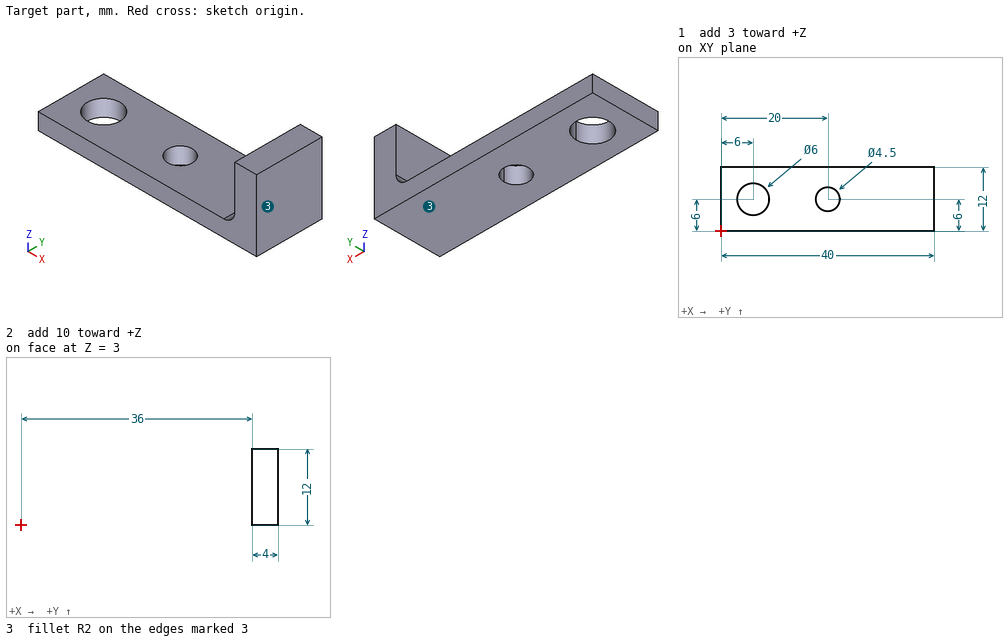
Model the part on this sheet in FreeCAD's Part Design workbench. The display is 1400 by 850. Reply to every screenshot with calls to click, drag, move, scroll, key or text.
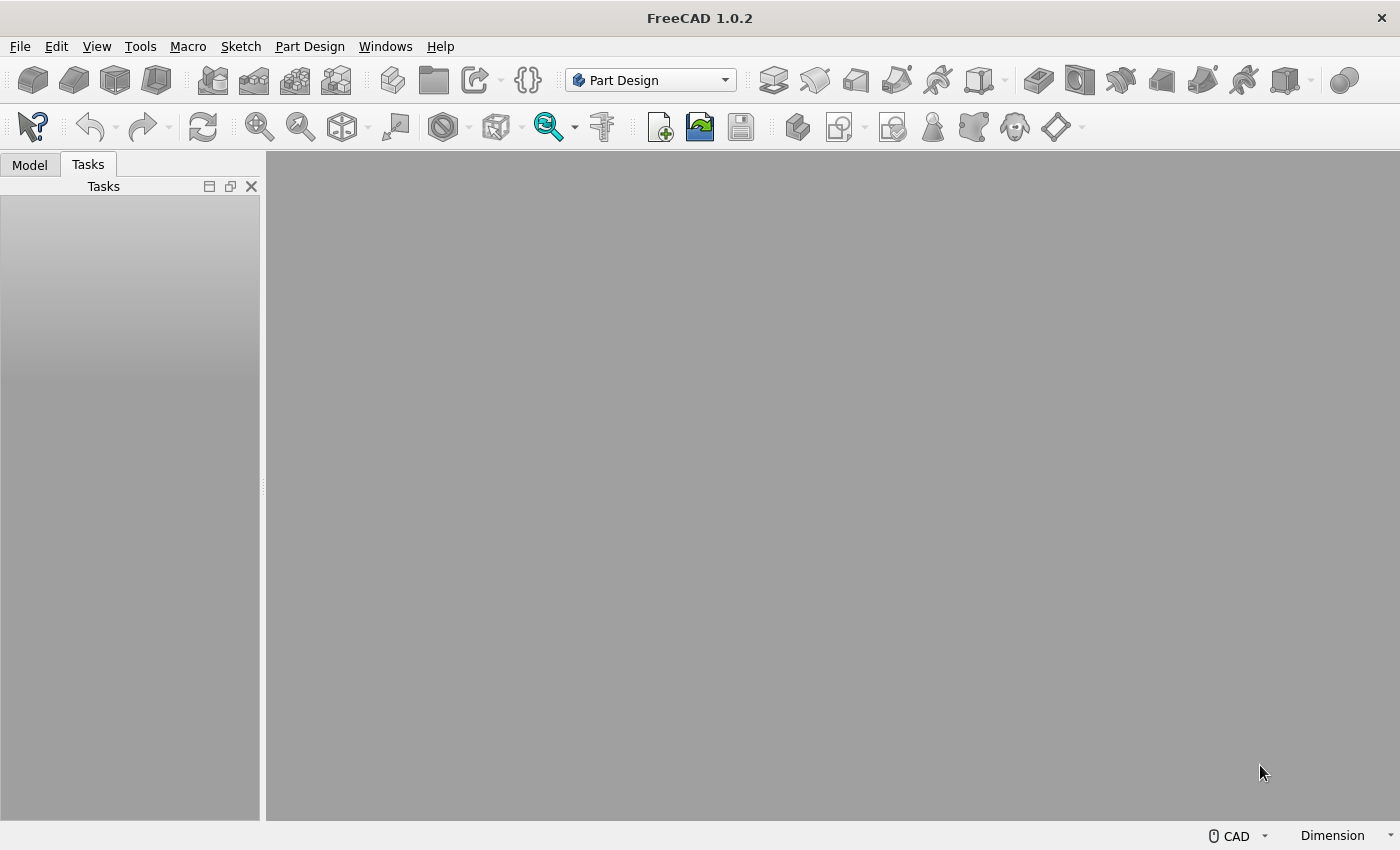
click(659, 128)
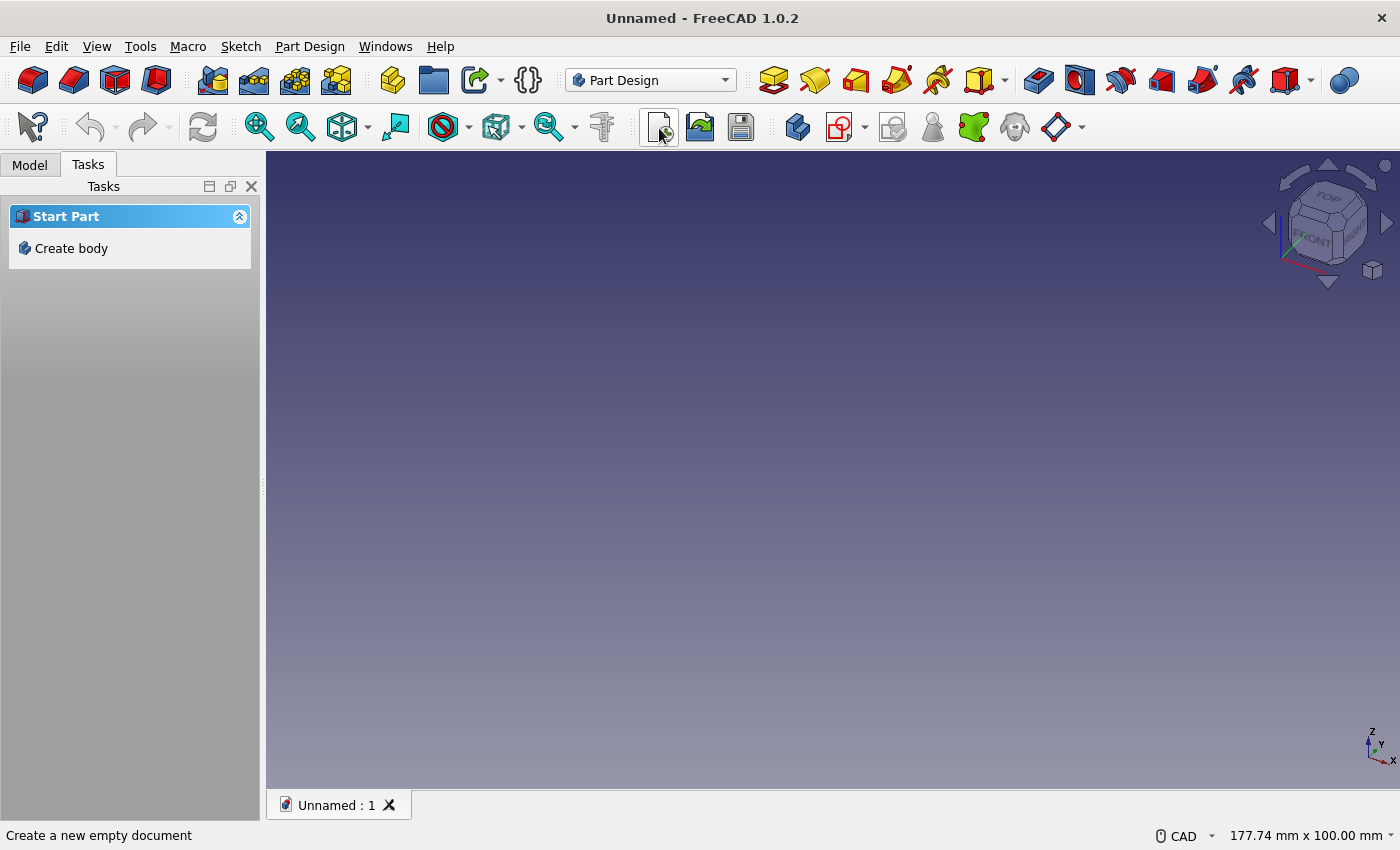
click(838, 128)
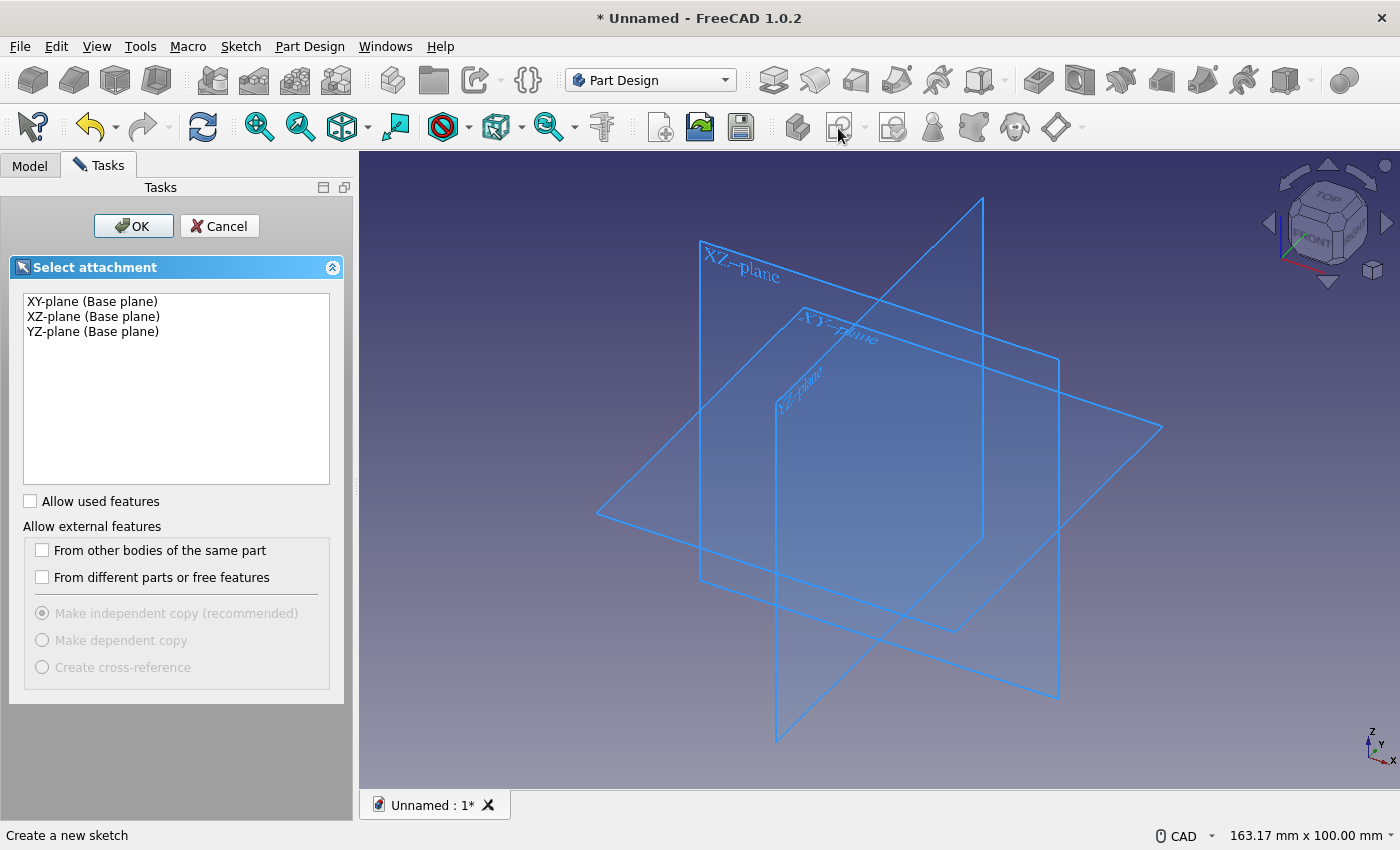
click(84, 302)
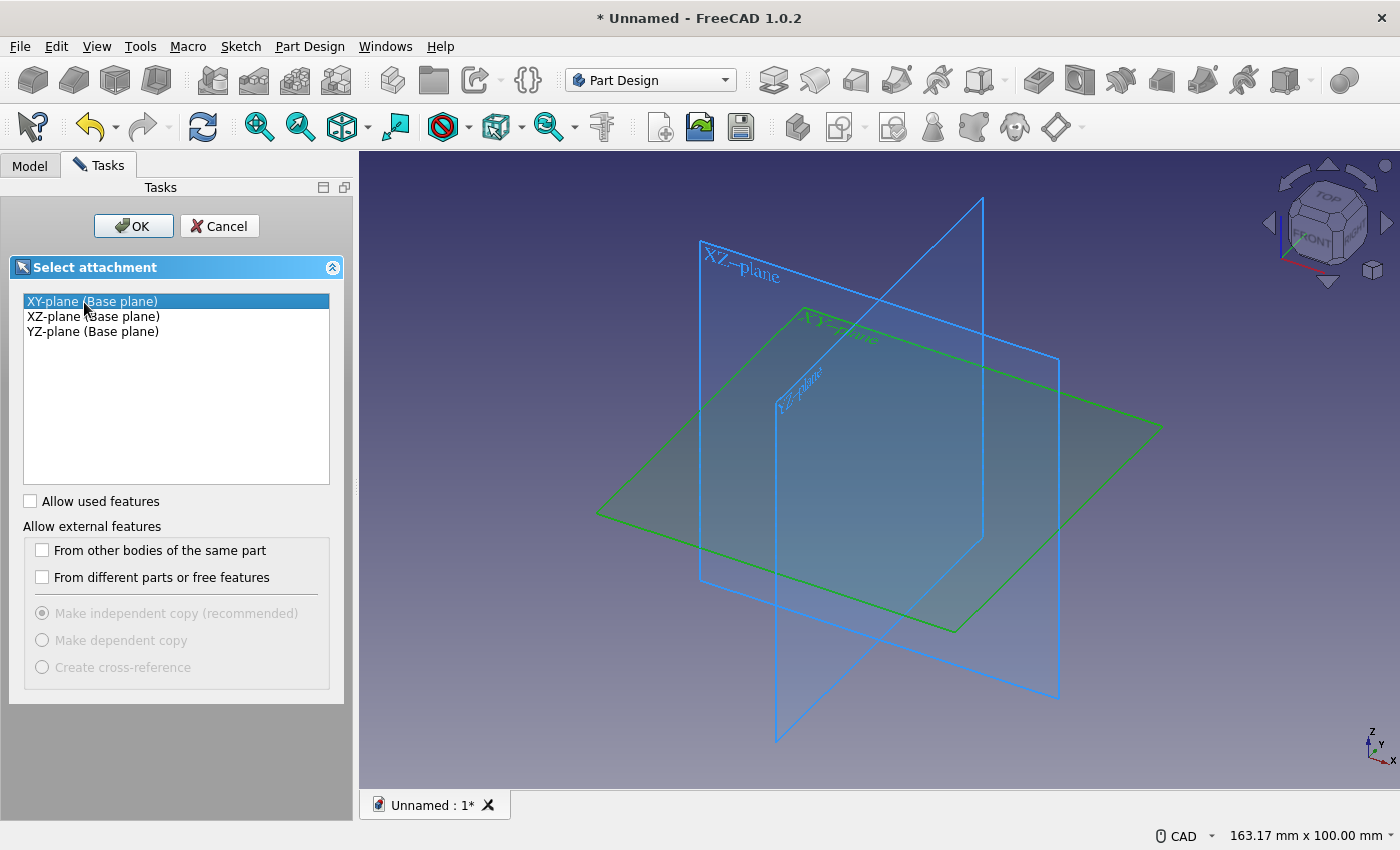
click(134, 226)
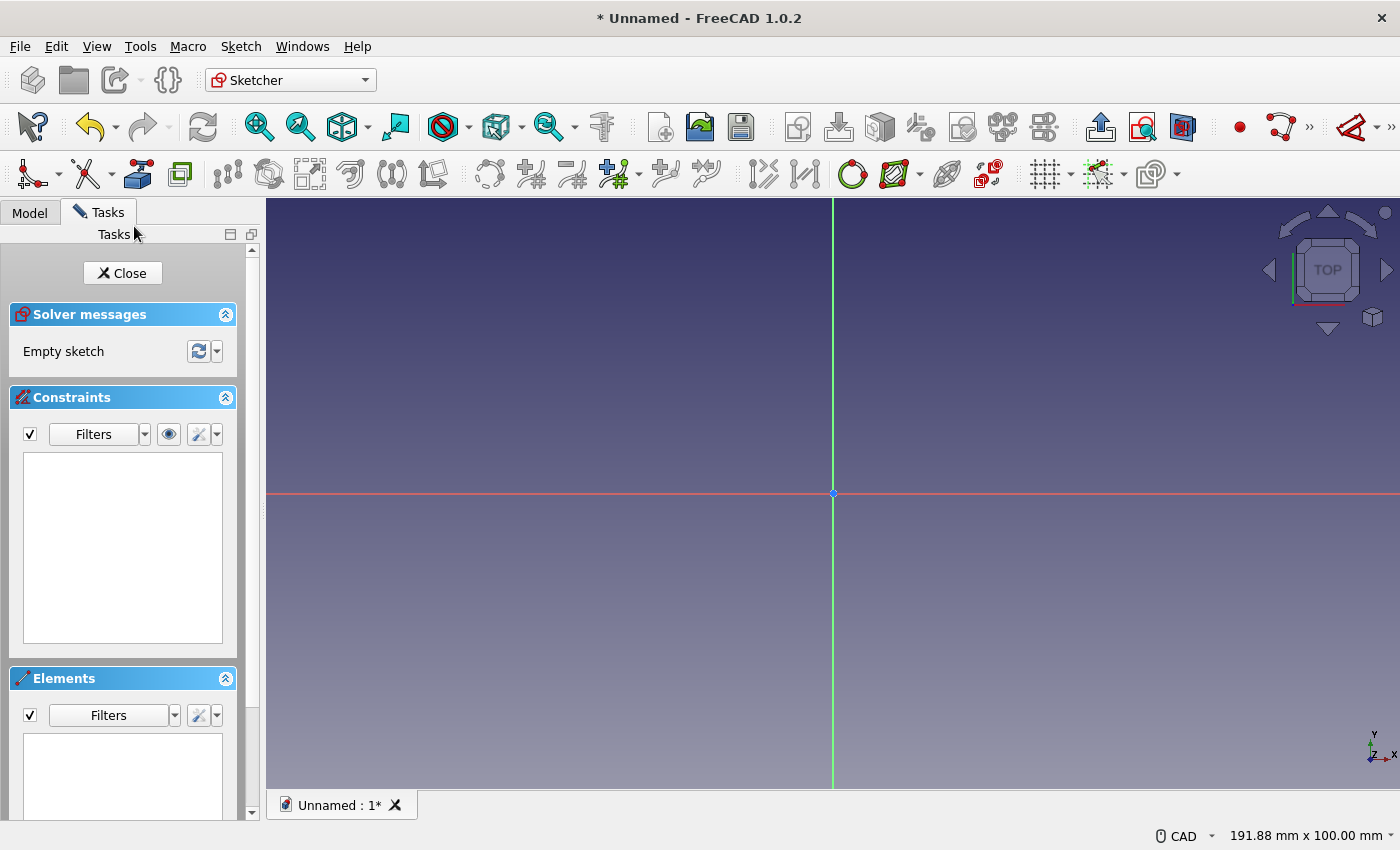
scroll(1060, 437, up, 5)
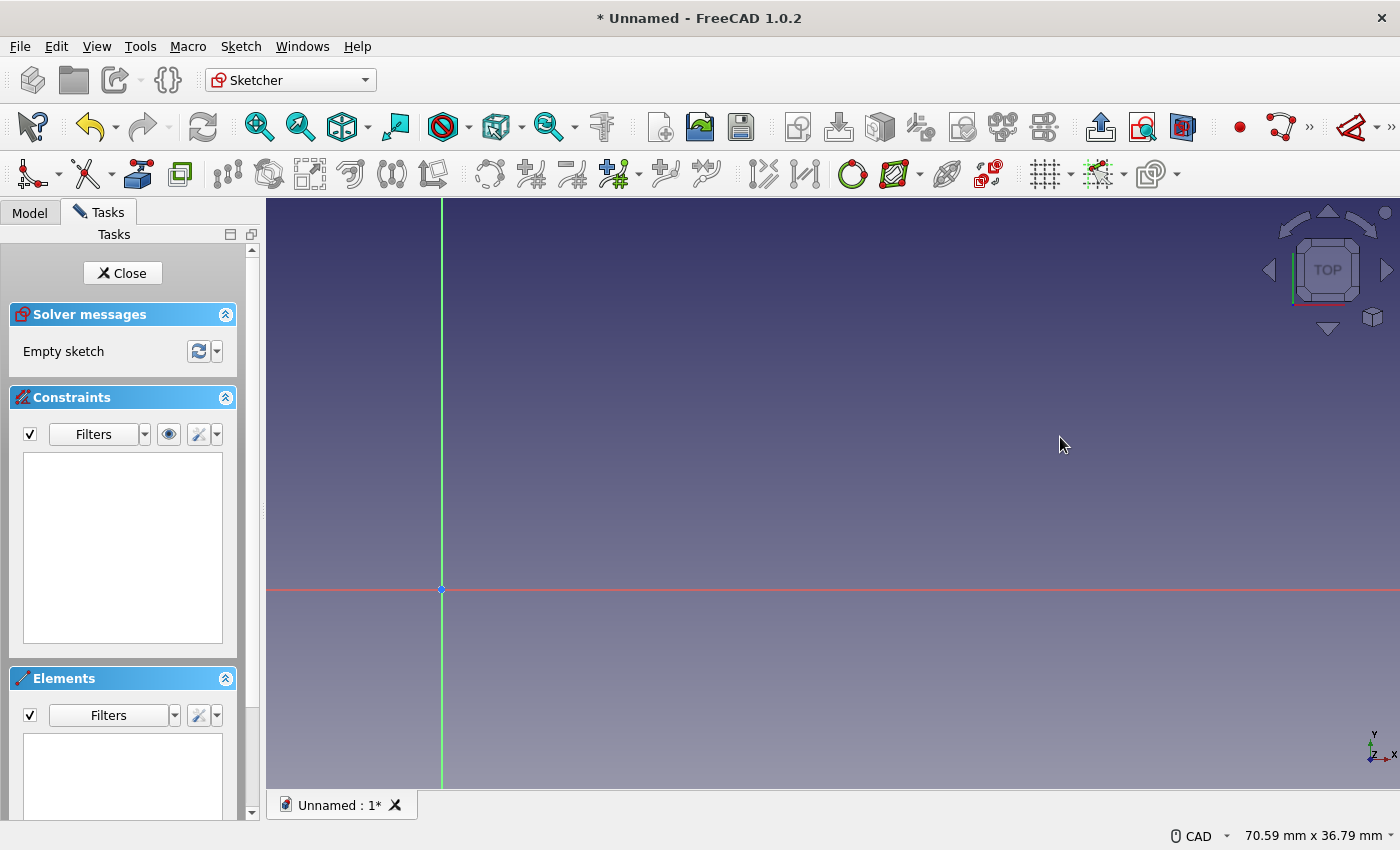
key(g)
key(r)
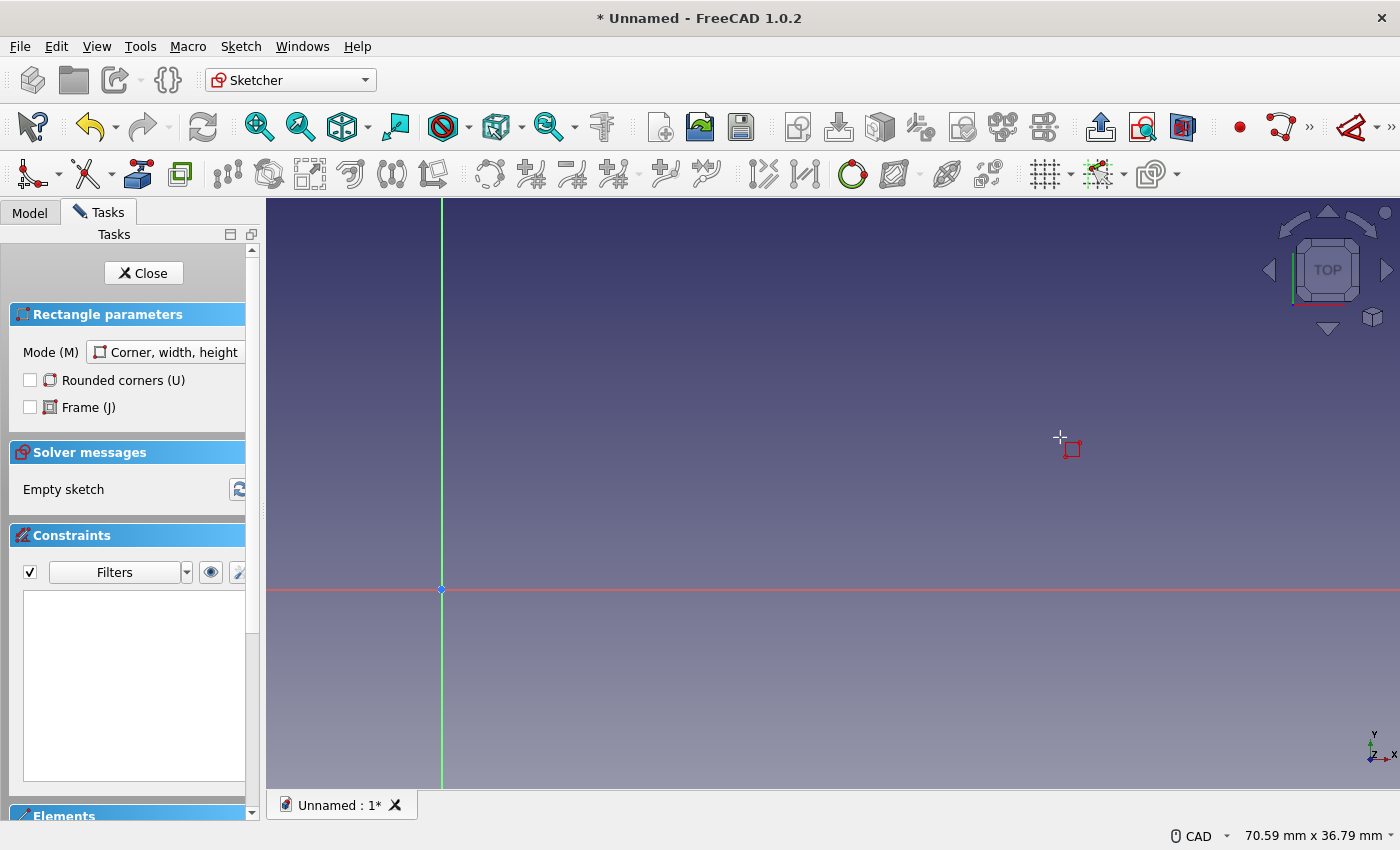
click(442, 590)
click(1084, 397)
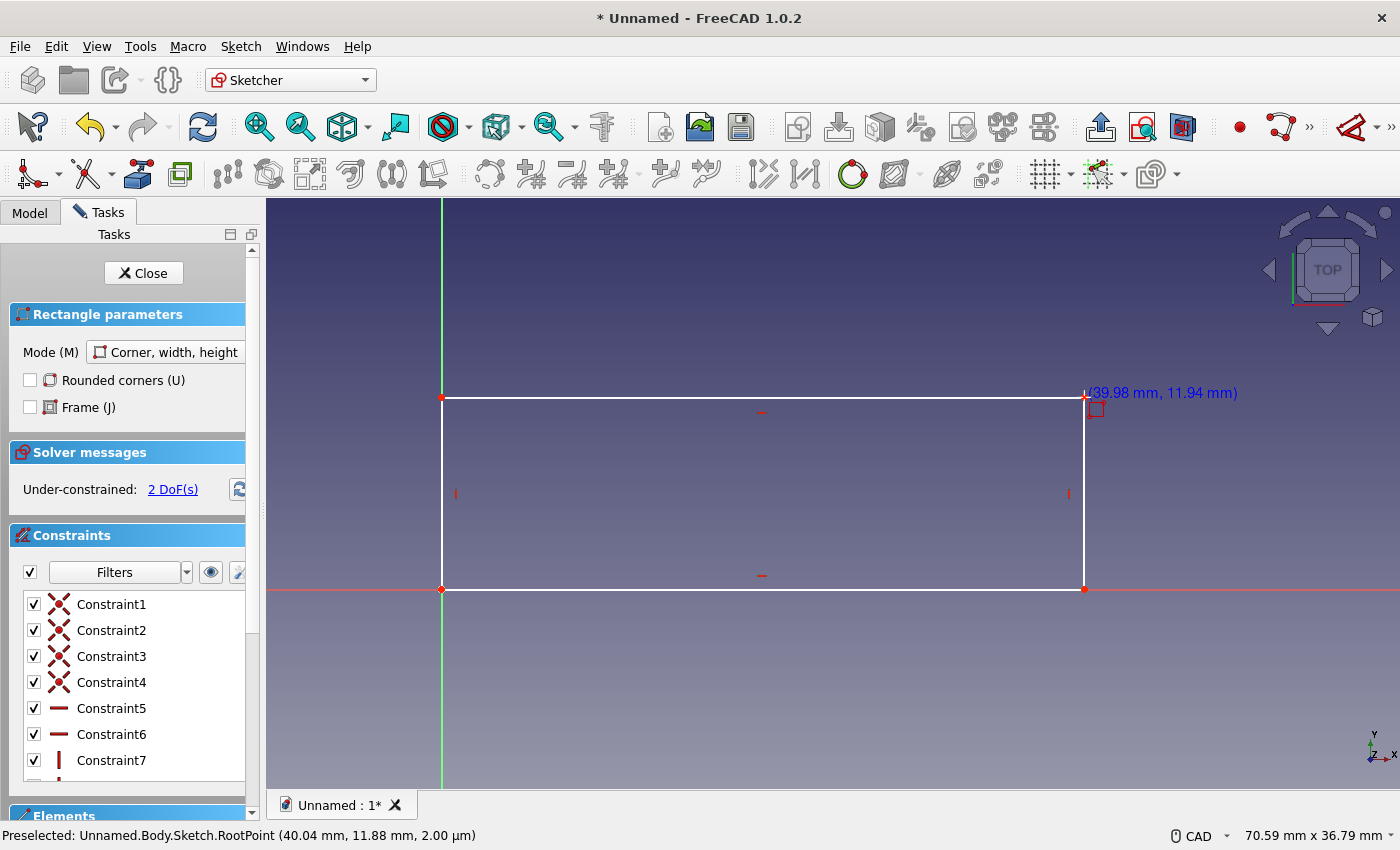
key(g)
key(c)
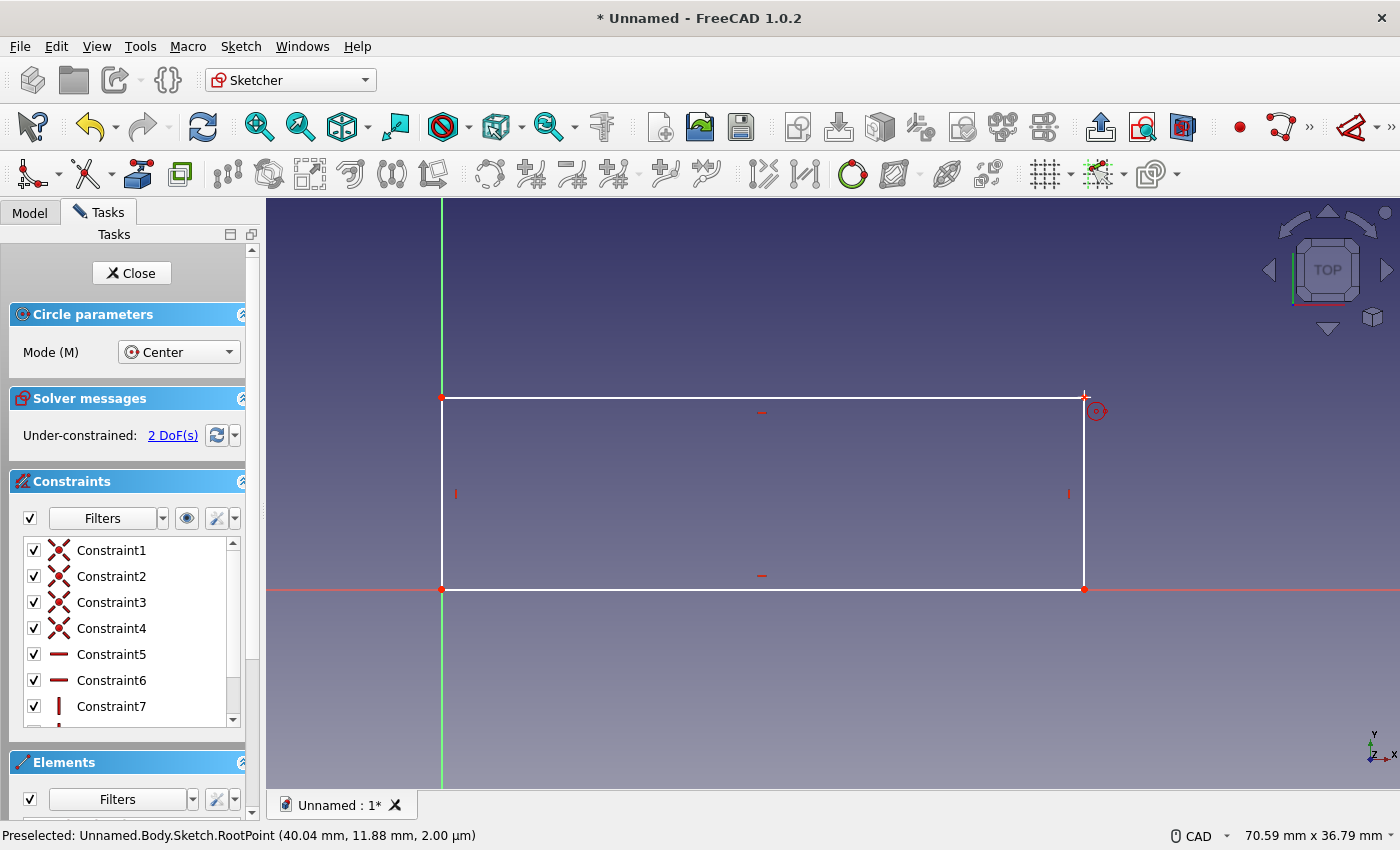
click(538, 493)
click(572, 459)